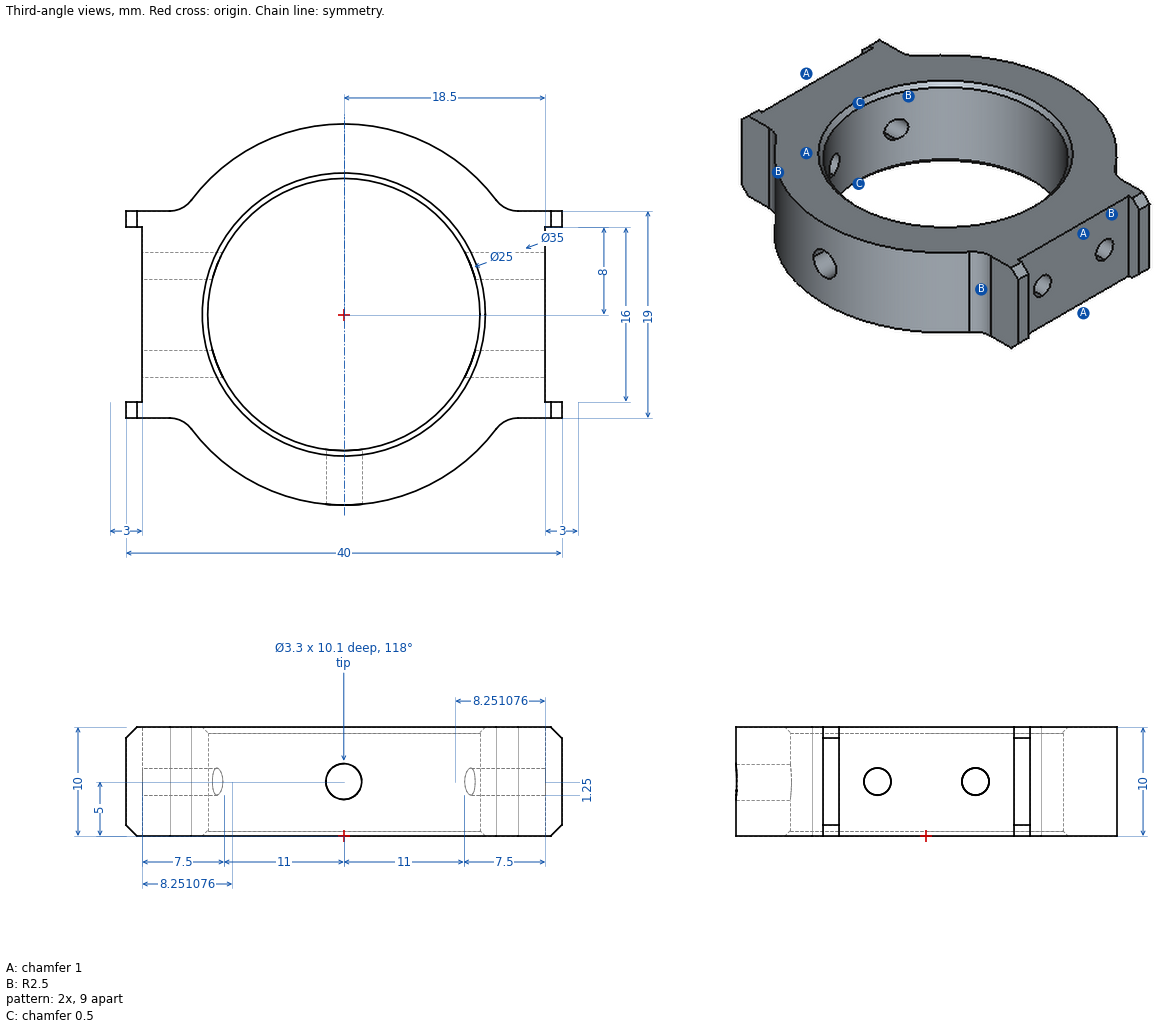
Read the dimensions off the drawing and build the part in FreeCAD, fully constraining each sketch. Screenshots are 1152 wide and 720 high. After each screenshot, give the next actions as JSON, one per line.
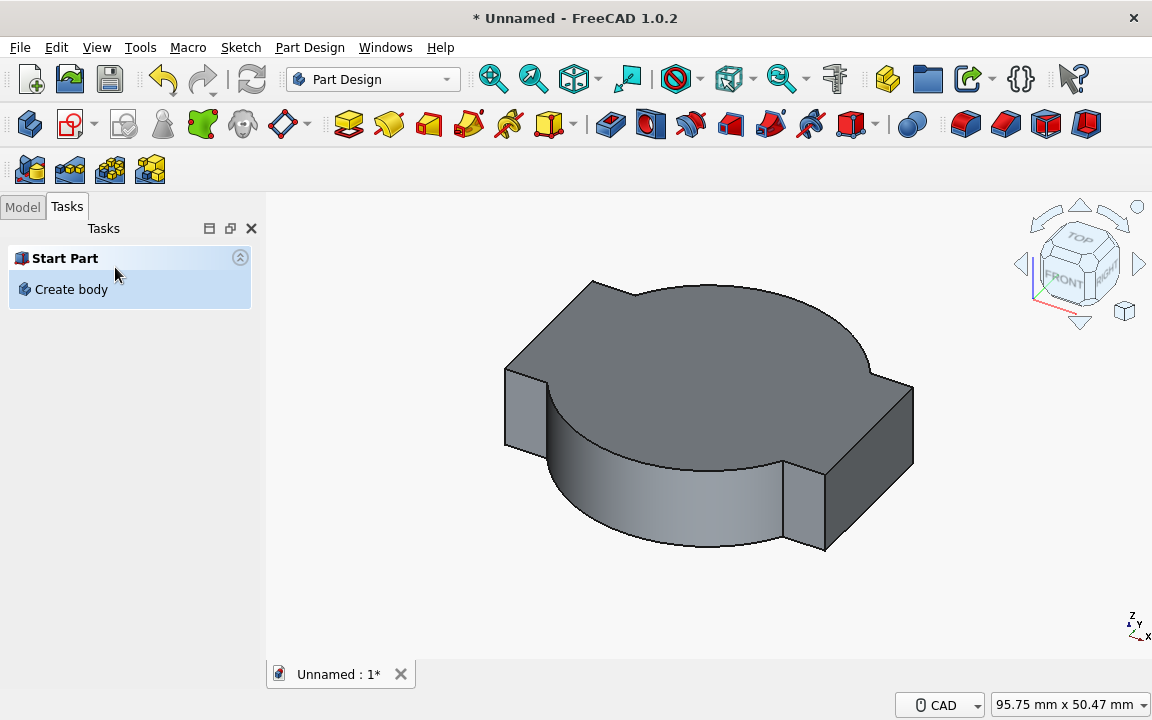
{"action": "left_click", "coordinate": [869, 430]}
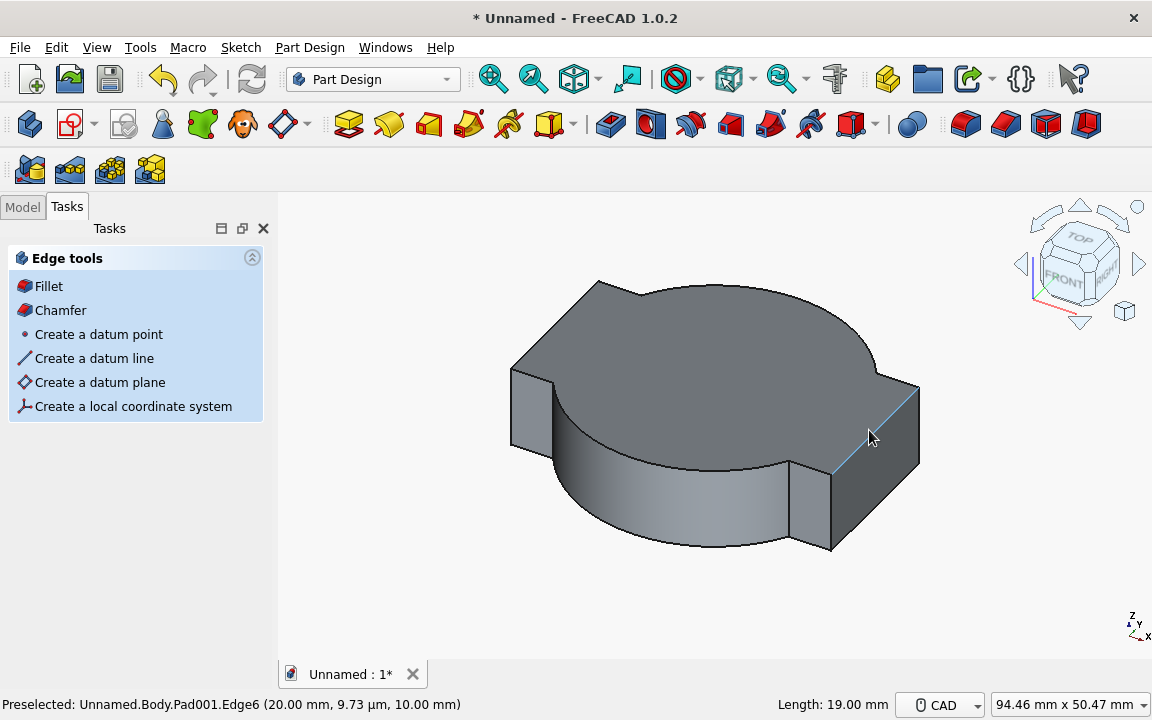
{"action": "key", "text": "0"}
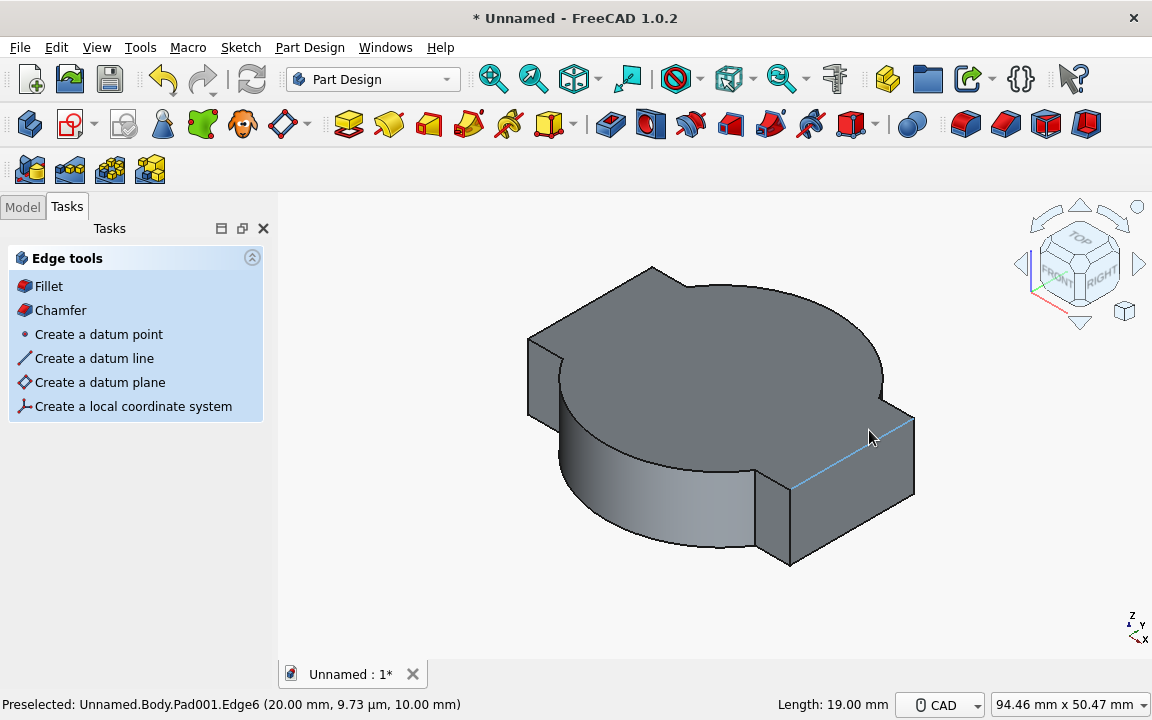
{"action": "key", "text": "2"}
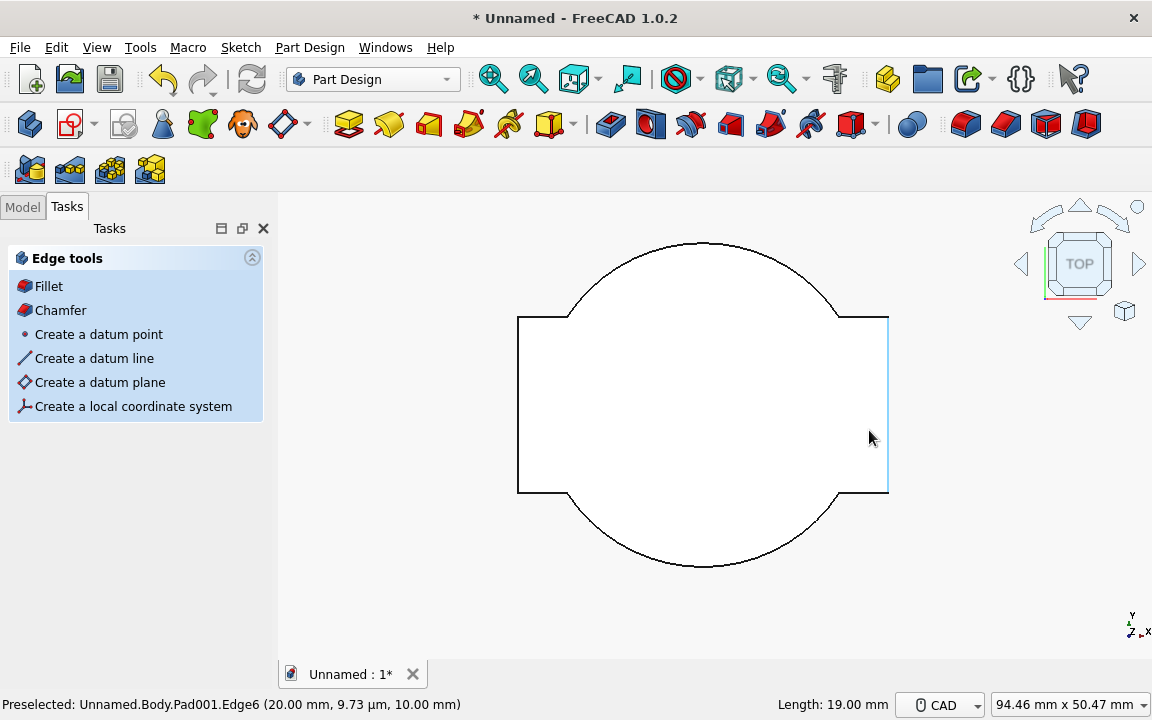
{"action": "left_click", "coordinate": [518, 404], "text": "ctrl"}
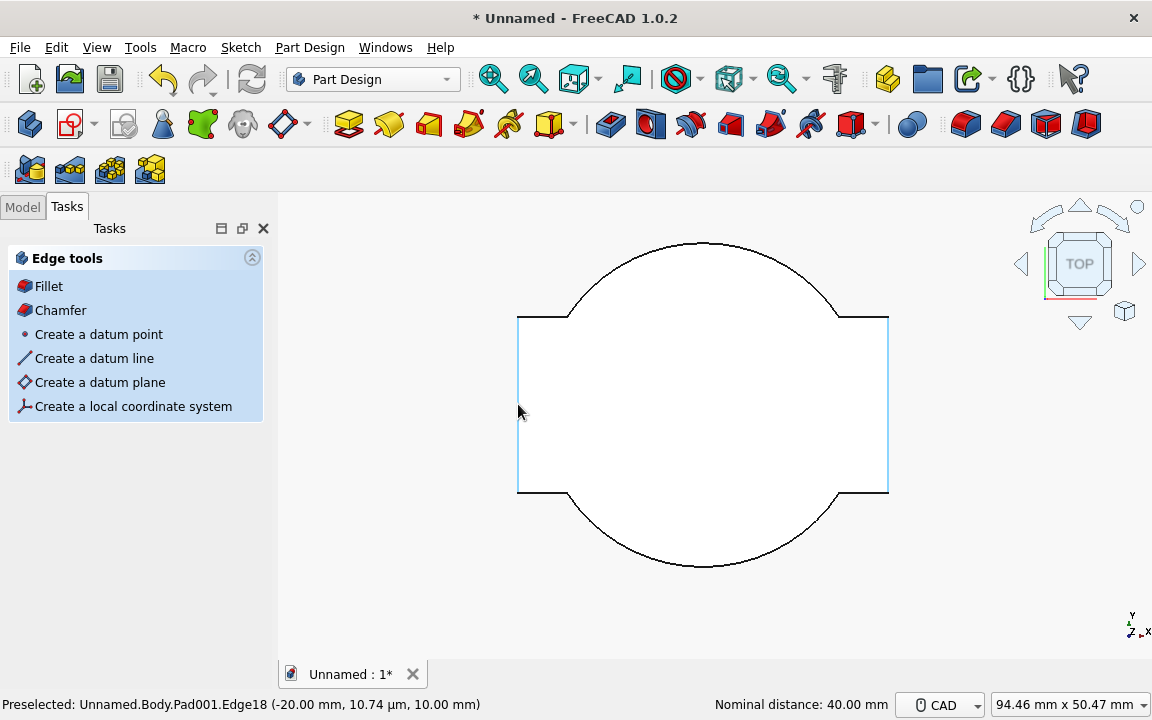
{"action": "key", "text": "1"}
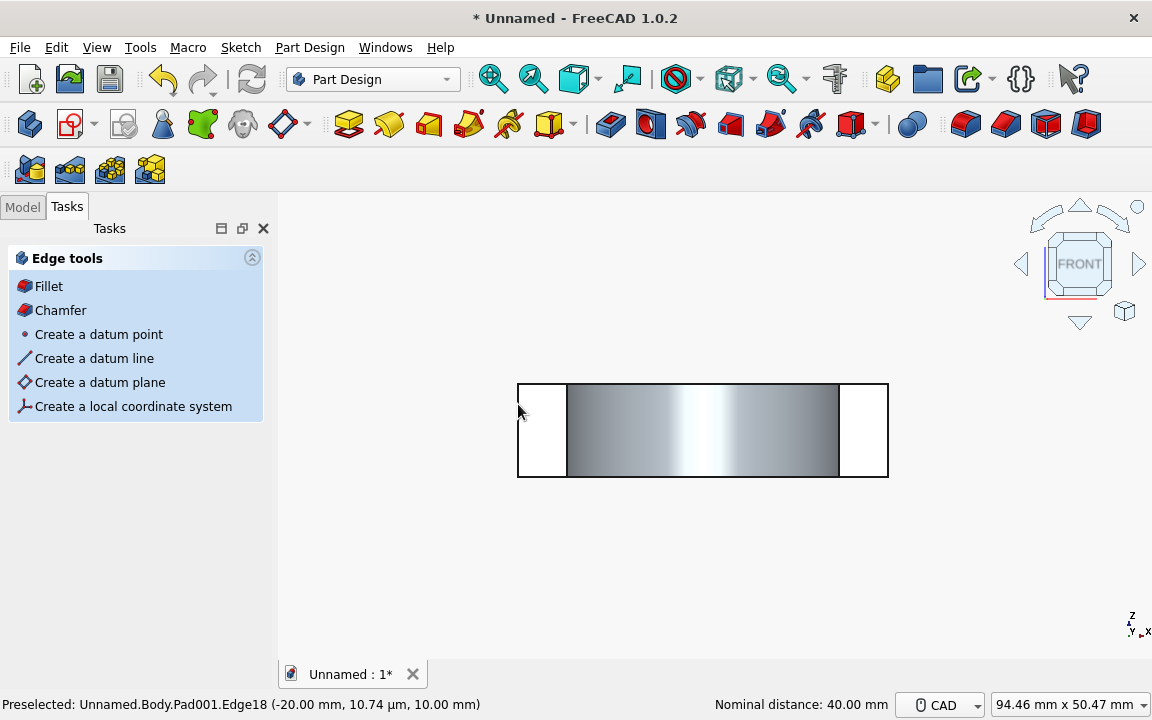
{"action": "left_click", "coordinate": [494, 80]}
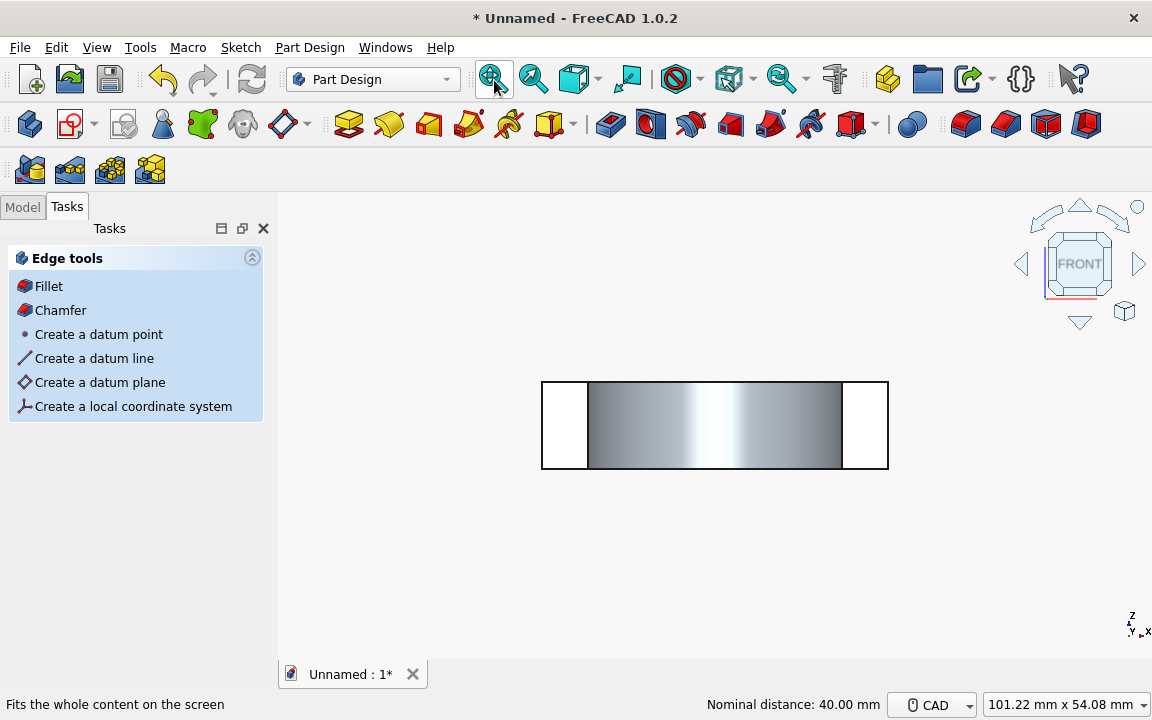
{"action": "key", "text": "3"}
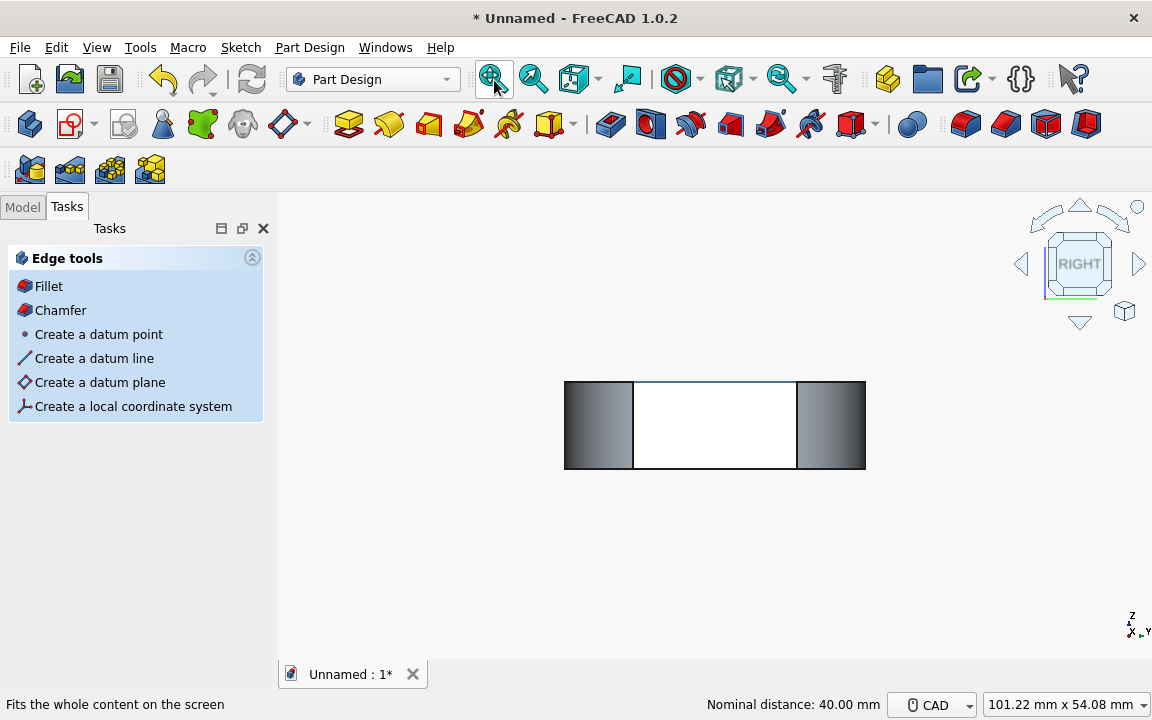
{"action": "left_click", "coordinate": [494, 80]}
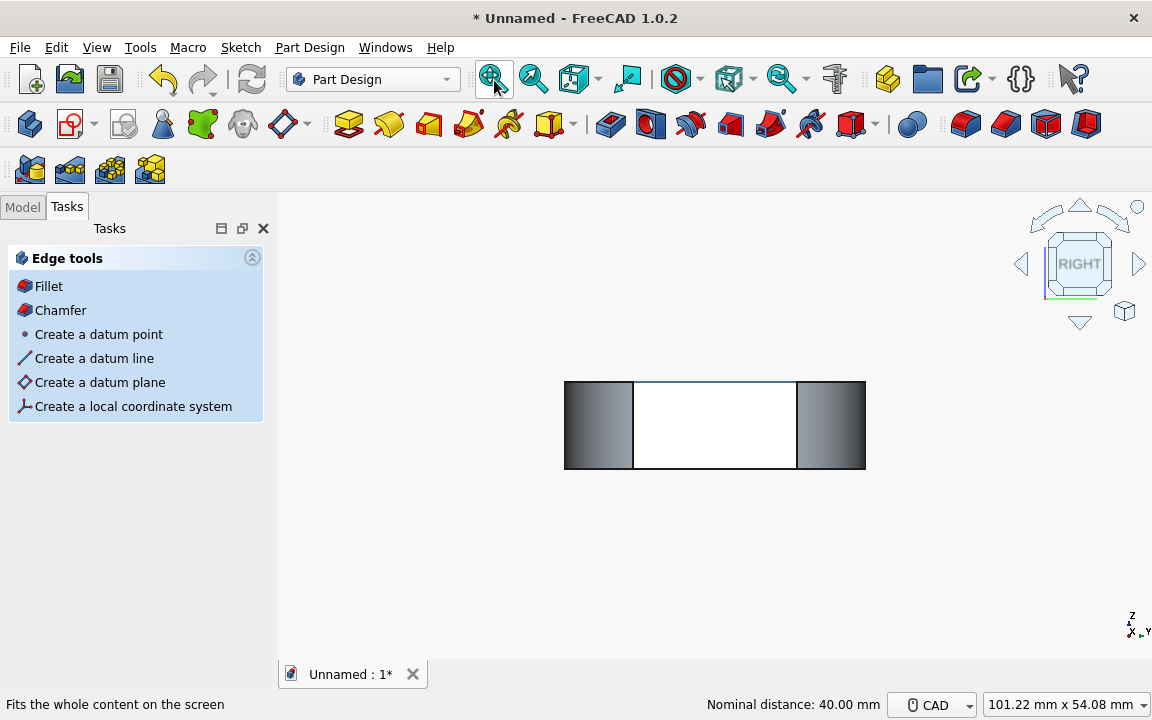
{"action": "left_click", "coordinate": [715, 468], "text": "ctrl"}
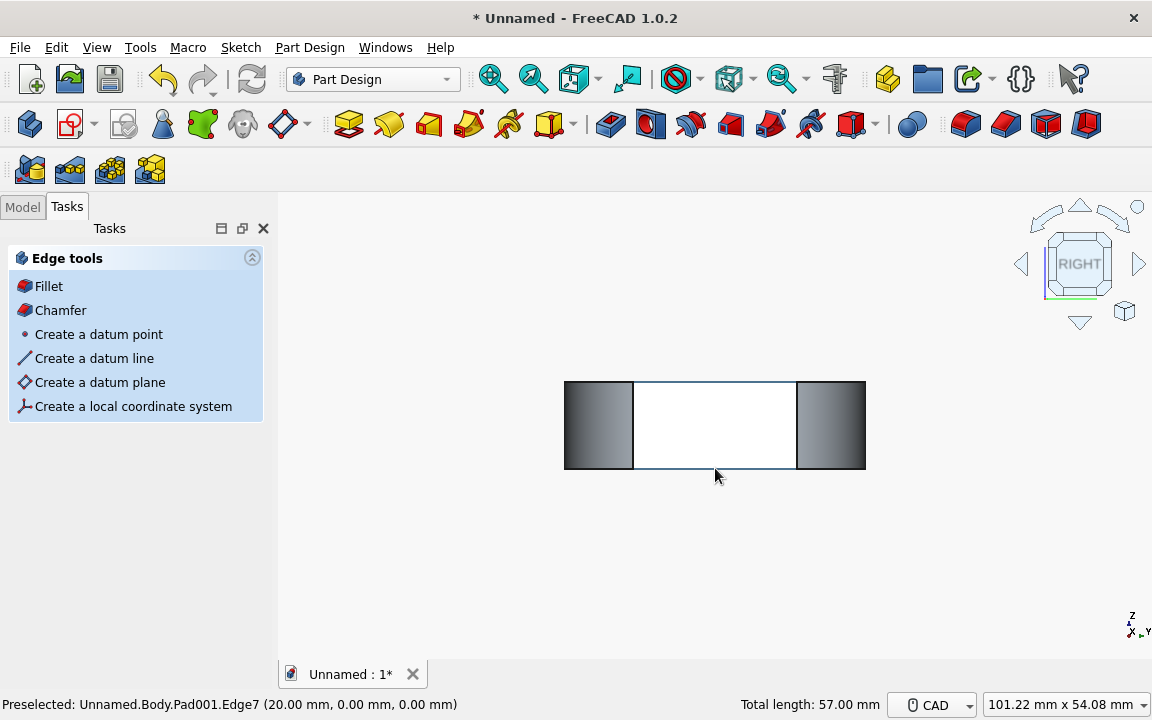
{"action": "key", "text": "5"}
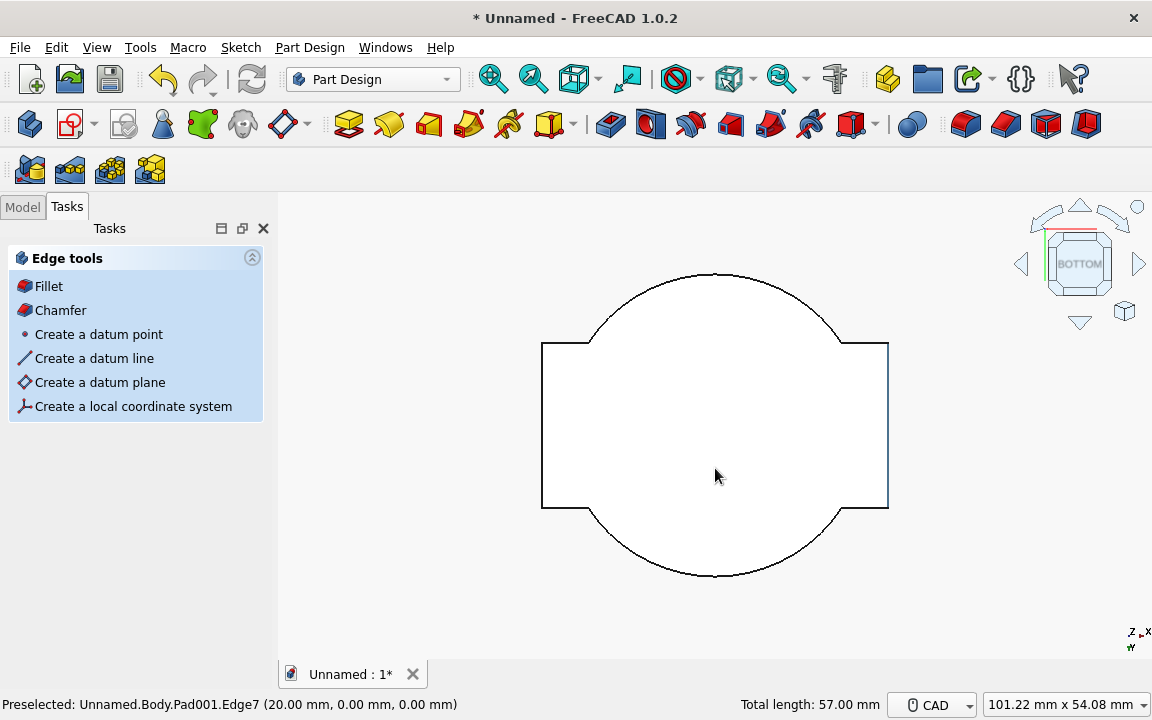
{"action": "left_click", "coordinate": [542, 424], "text": "ctrl"}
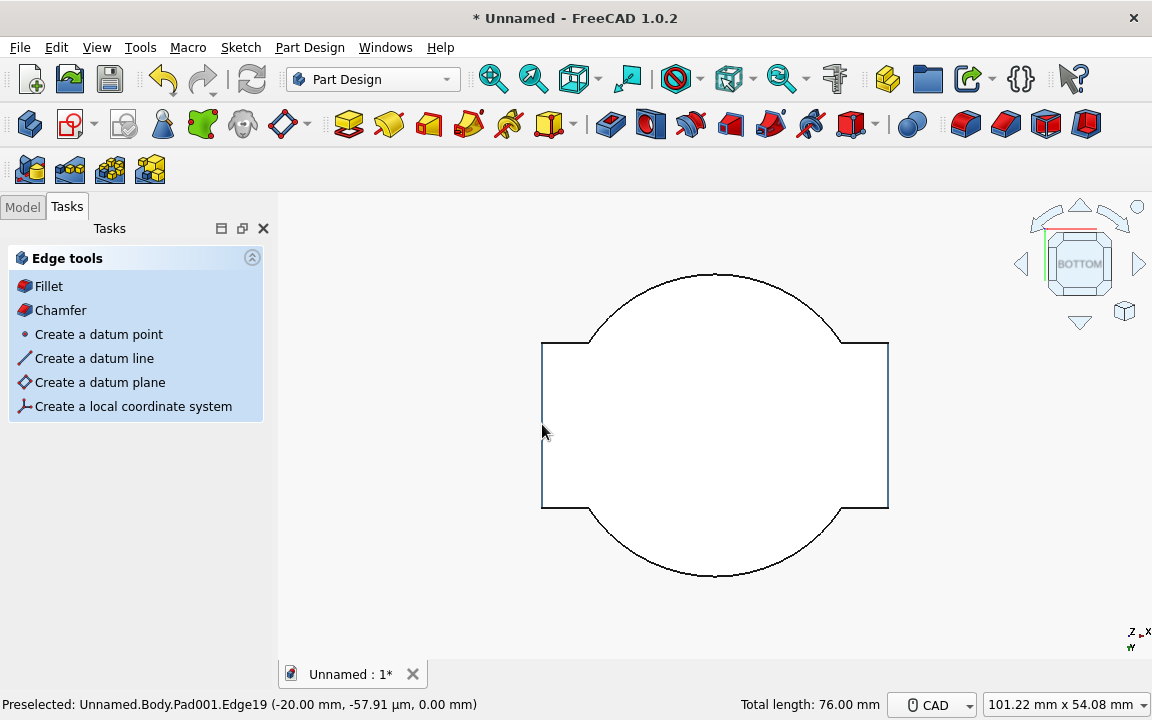
{"action": "left_click", "coordinate": [1006, 124]}